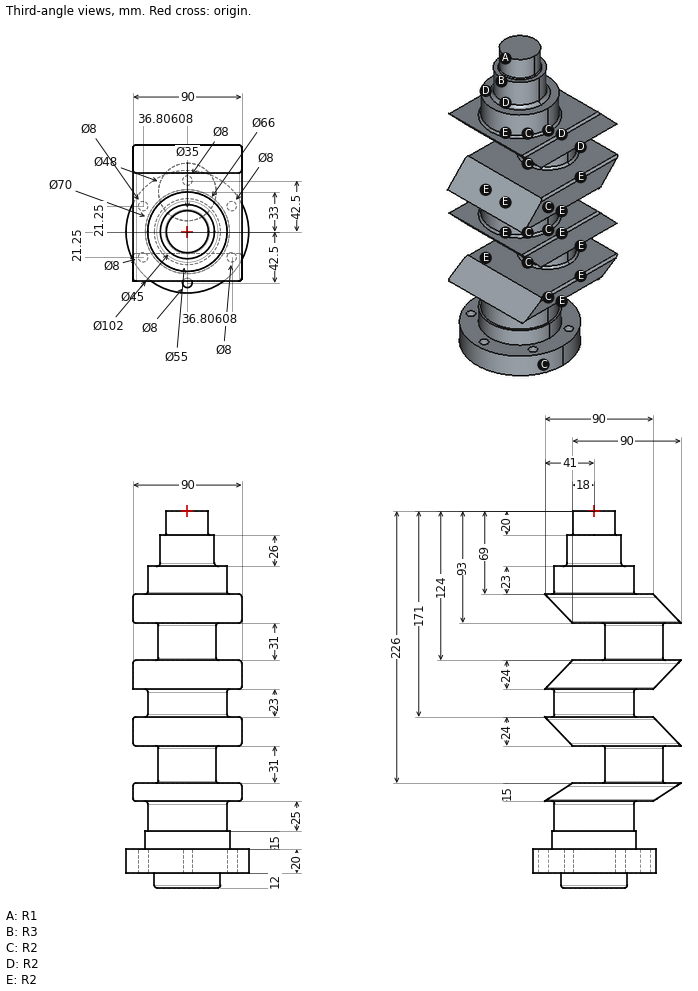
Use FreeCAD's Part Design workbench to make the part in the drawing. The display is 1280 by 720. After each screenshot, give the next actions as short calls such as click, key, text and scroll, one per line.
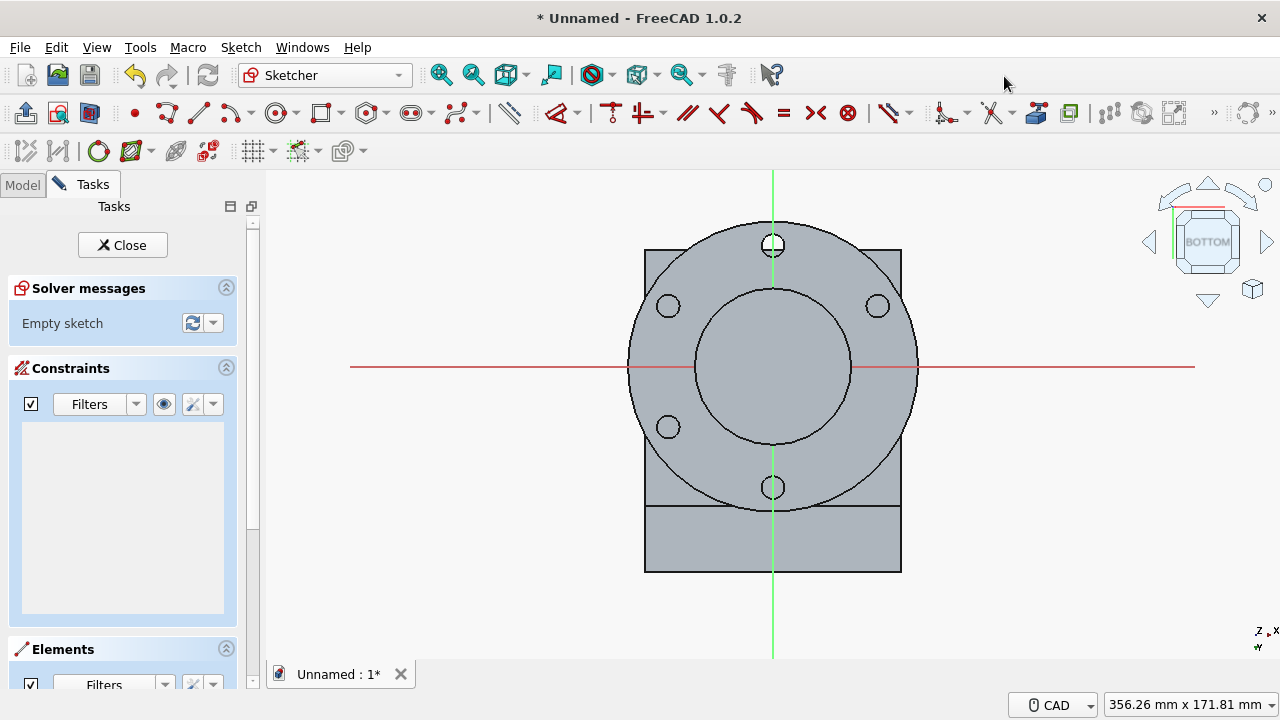
click(90, 114)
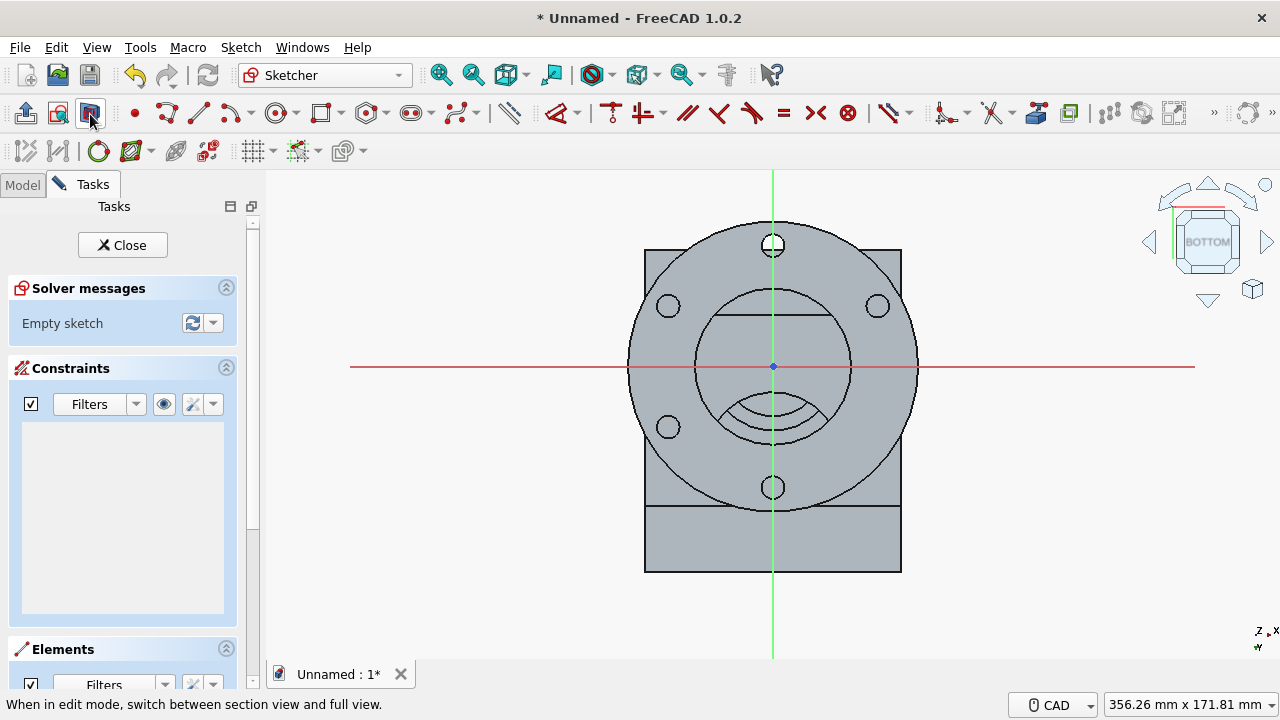
scroll(892, 428, up, 13)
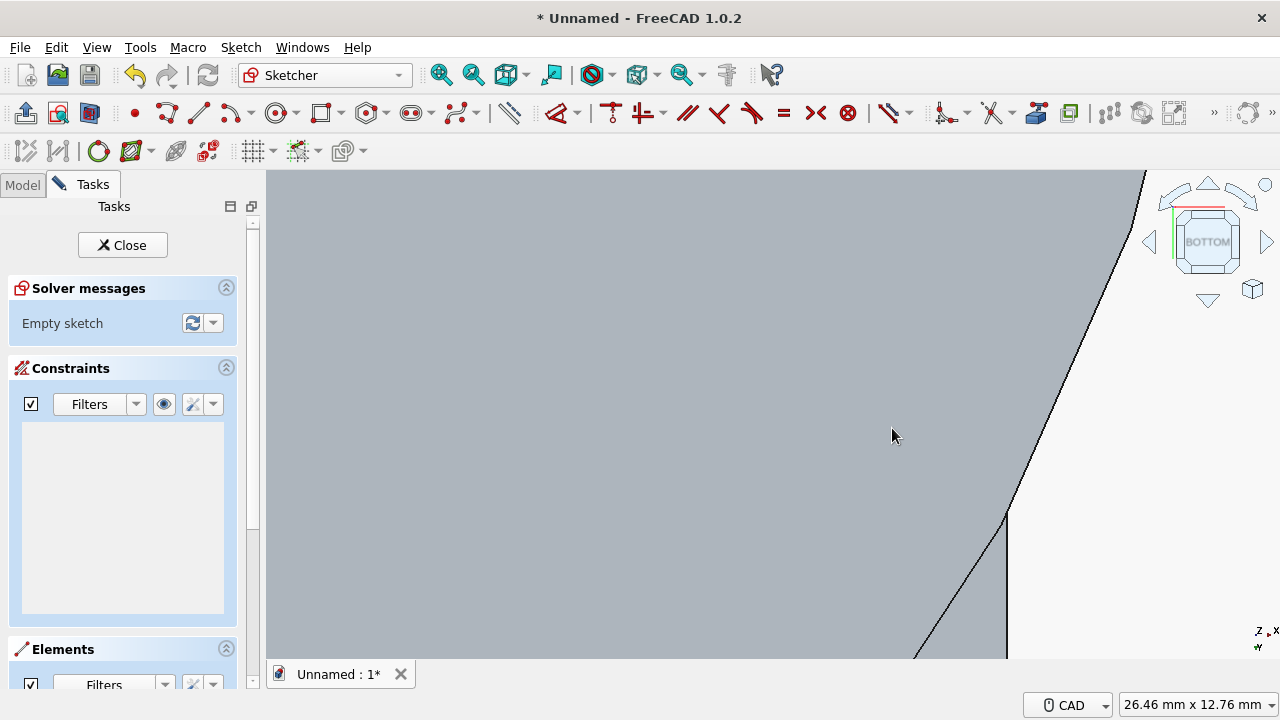
click(276, 114)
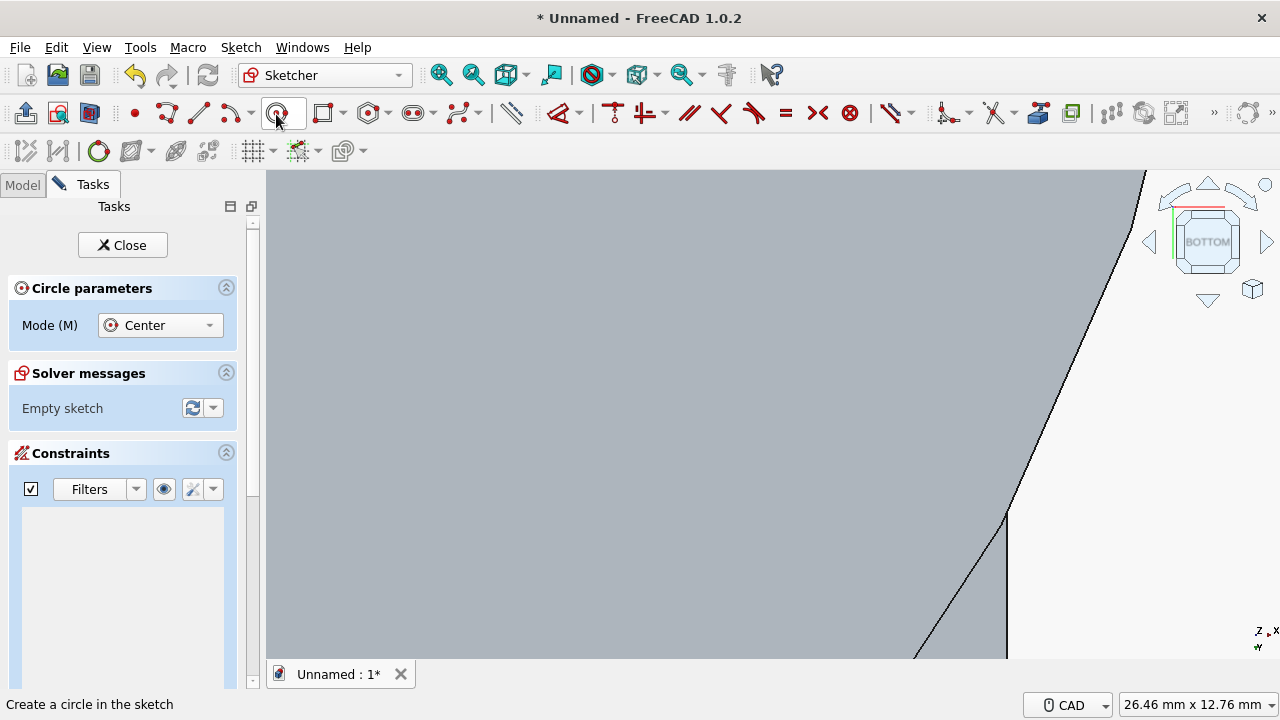
click(693, 409)
move(801, 301)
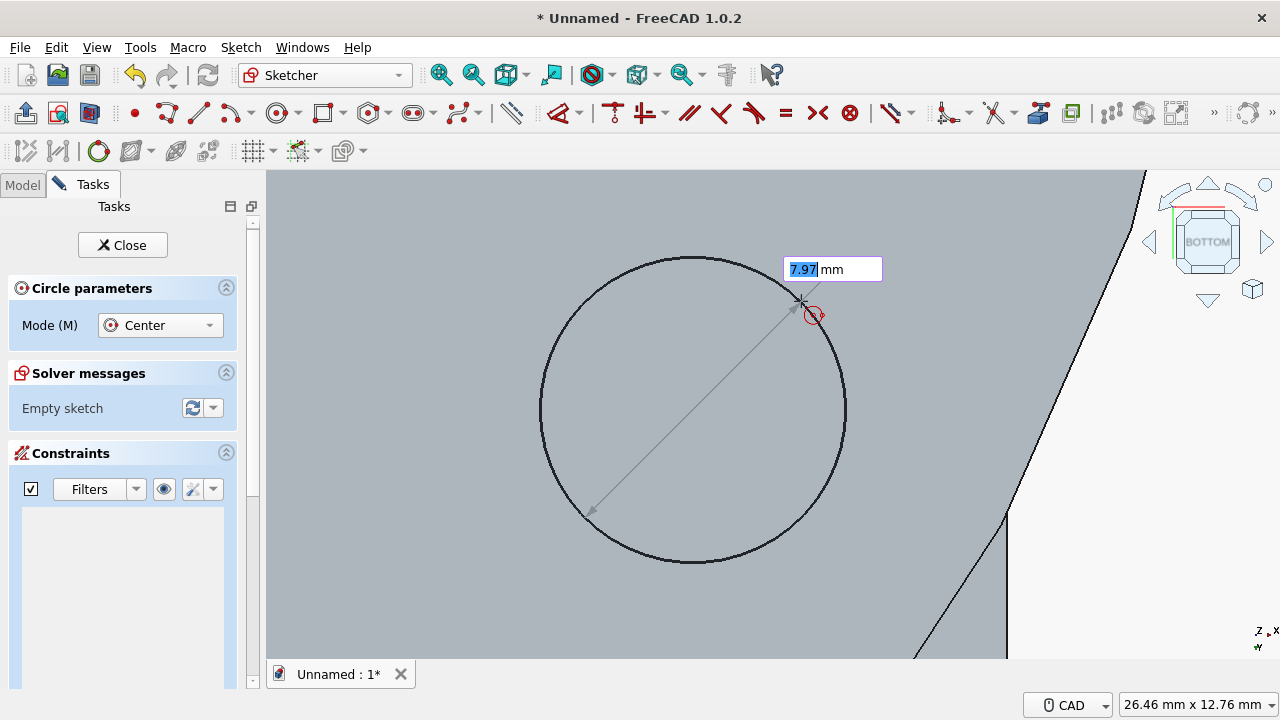
text(8)
key(Return)
key(Escape)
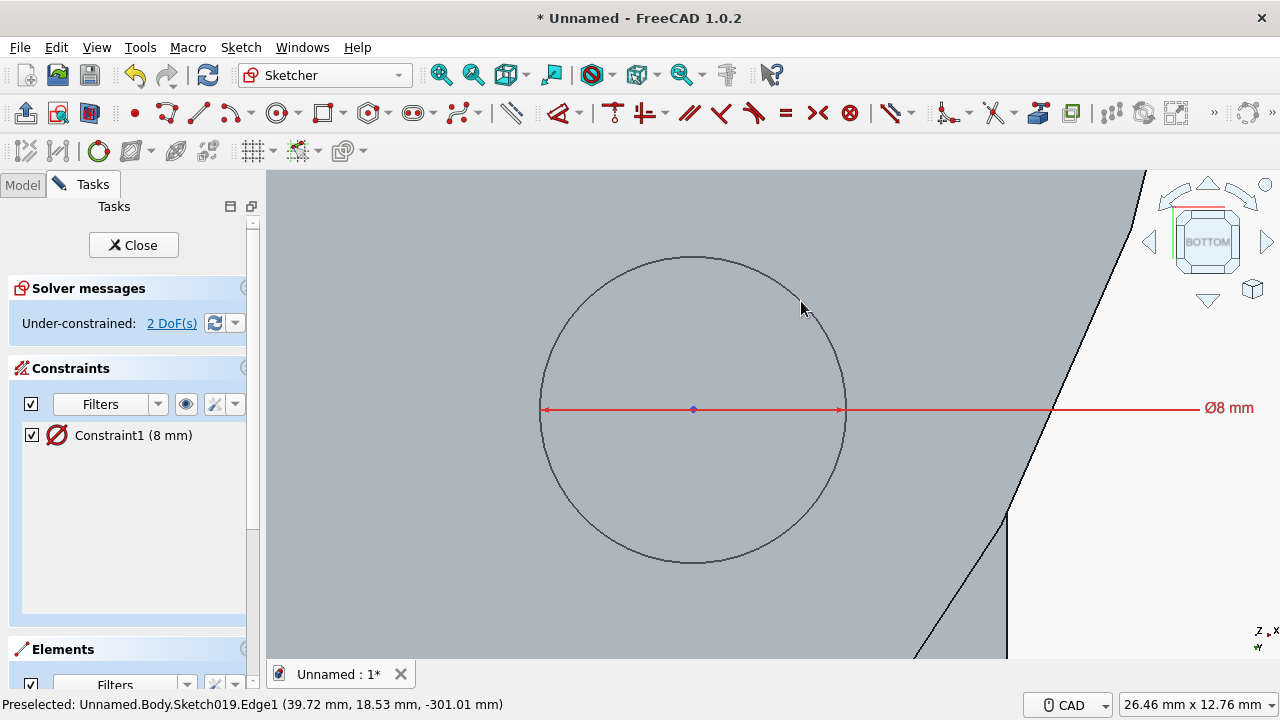
click(558, 114)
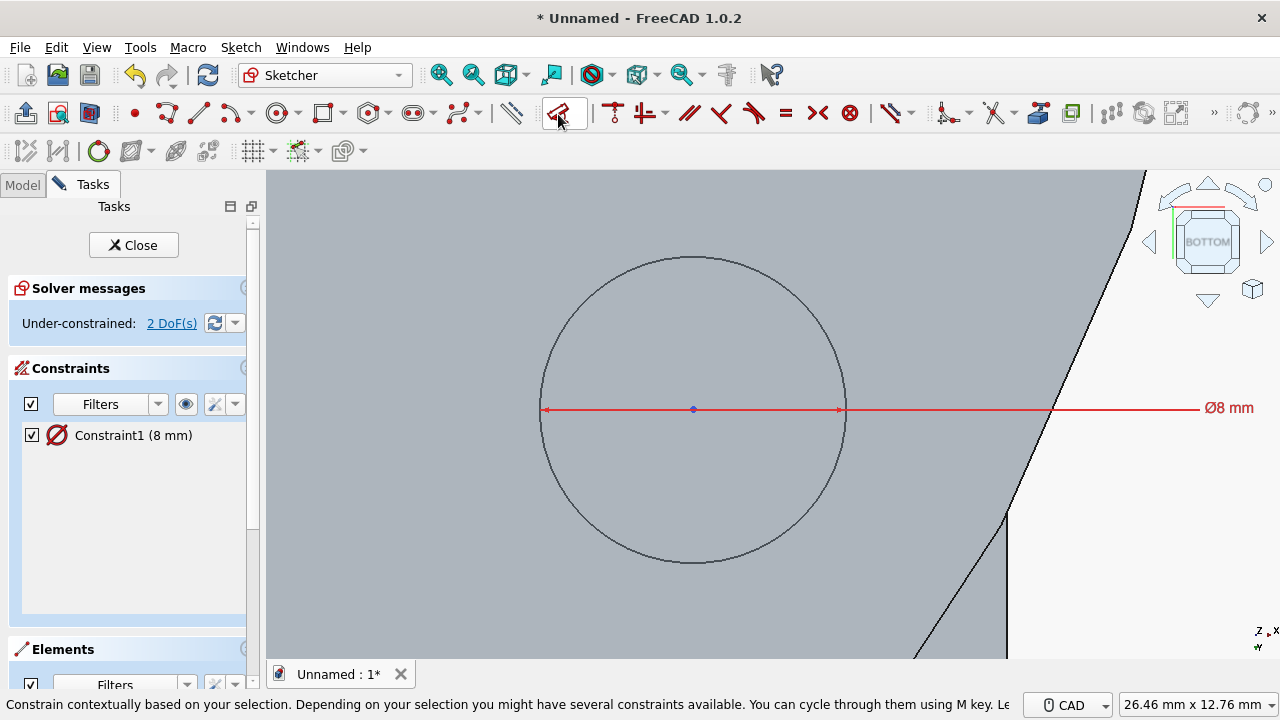
click(693, 410)
click(727, 304)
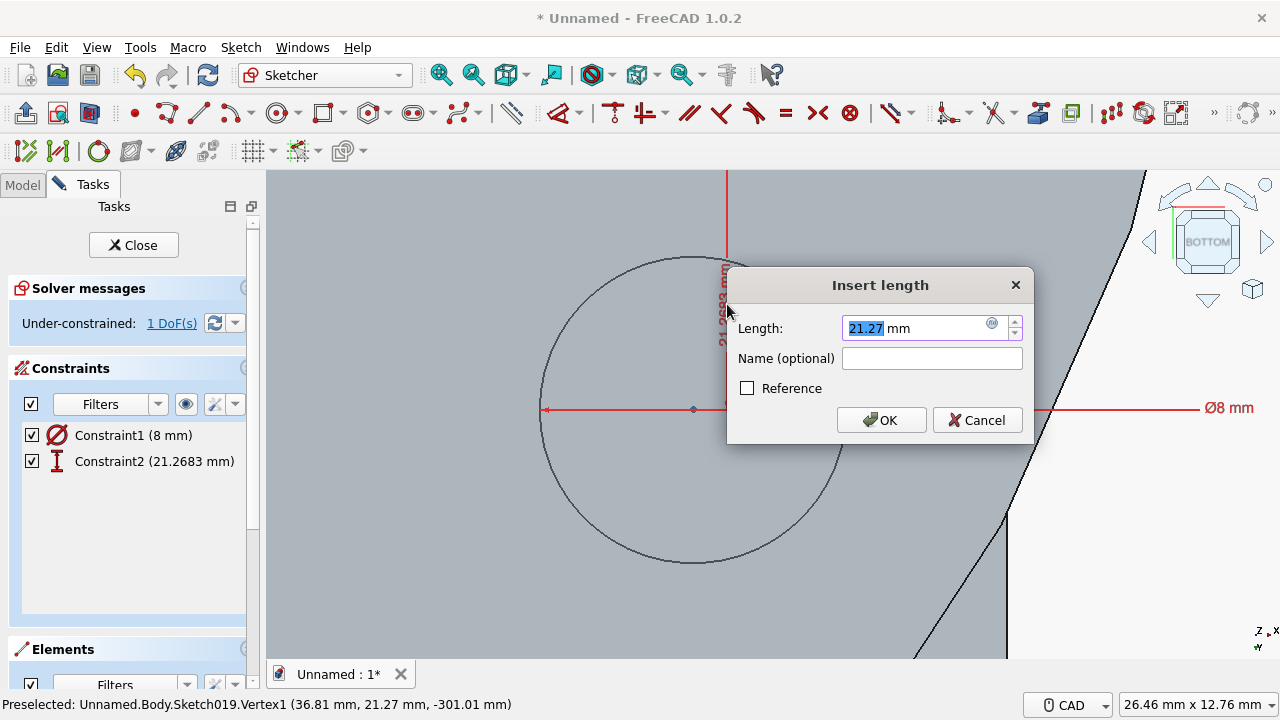
text(21.25)
key(Return)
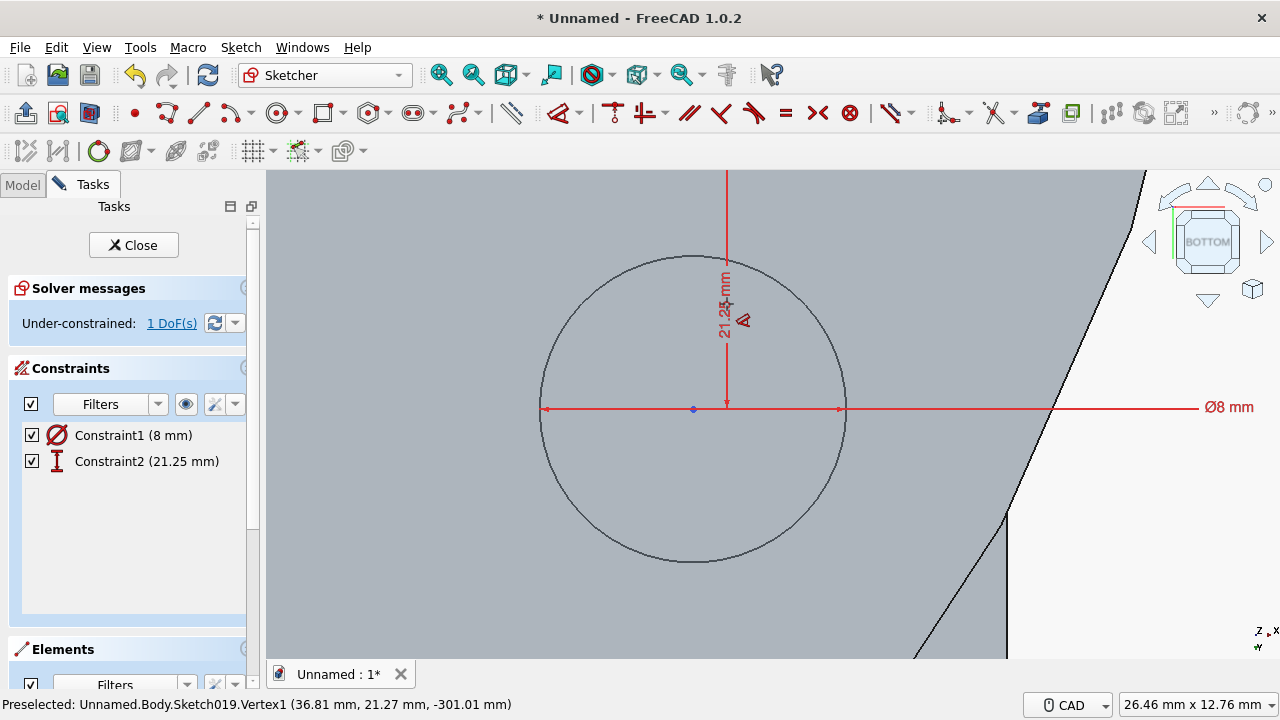
click(693, 409)
click(494, 443)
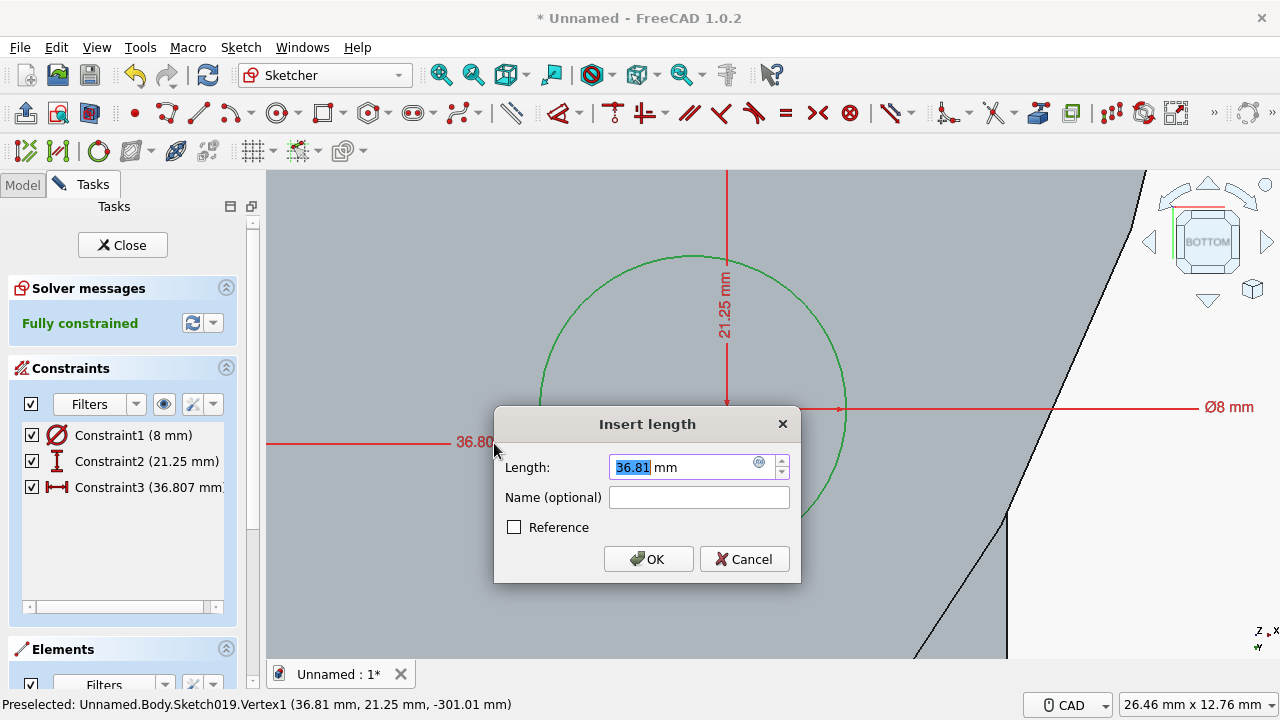
text(36.80608)
key(Return)
key(Escape)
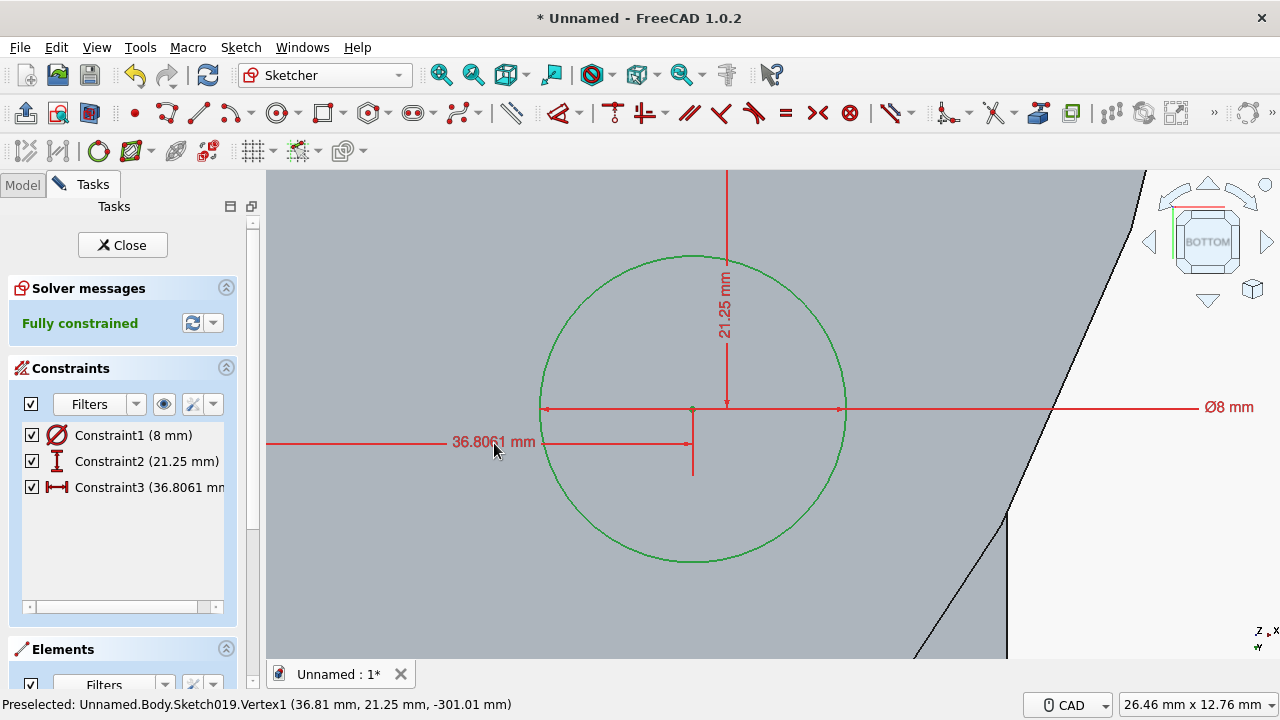
click(123, 245)